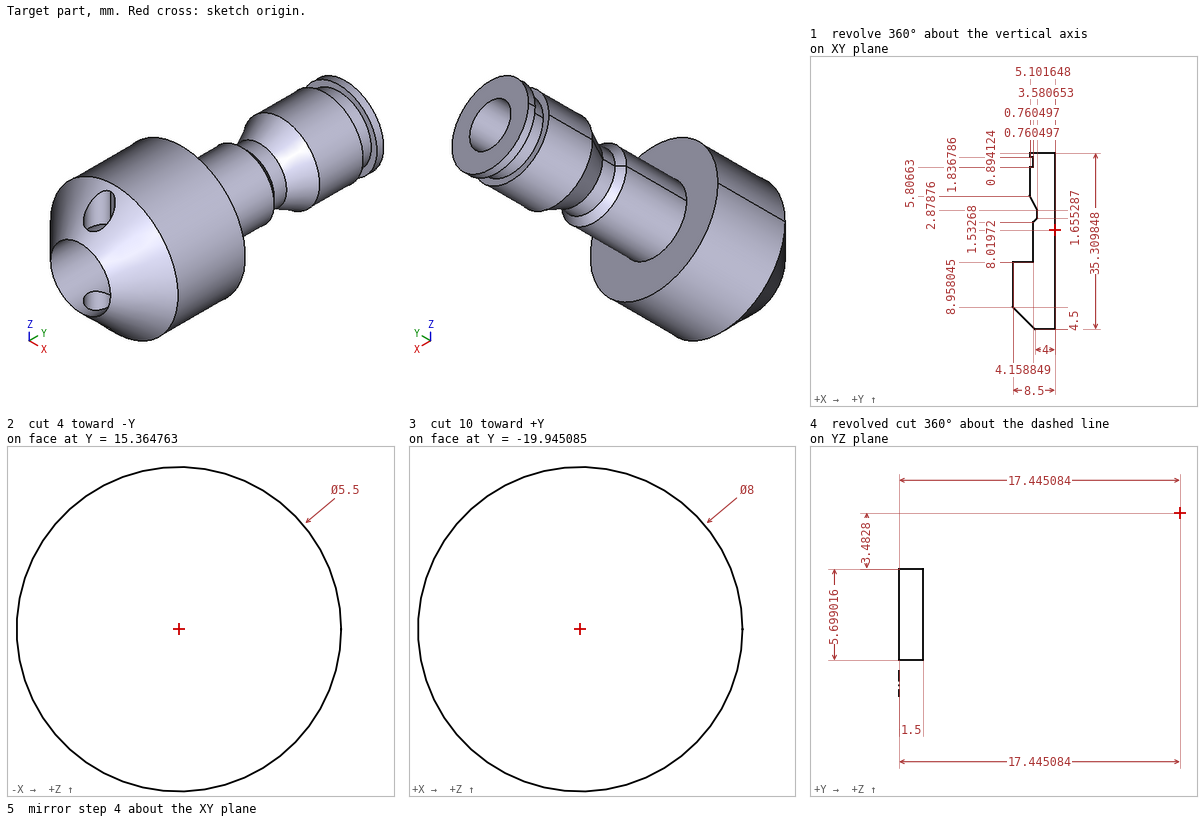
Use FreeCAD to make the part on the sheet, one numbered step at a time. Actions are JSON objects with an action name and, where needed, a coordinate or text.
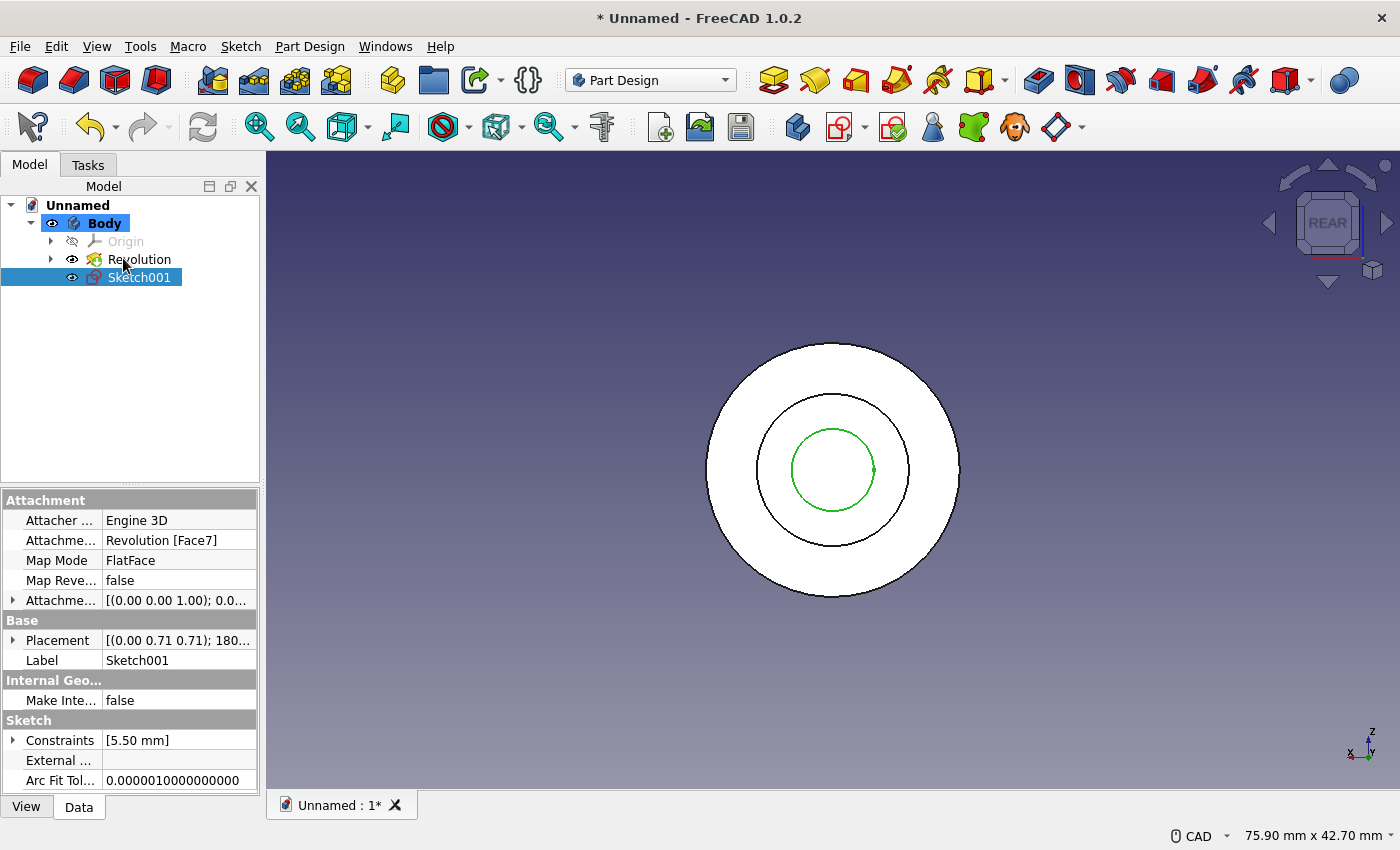
{"action": "left_click", "coordinate": [1039, 80]}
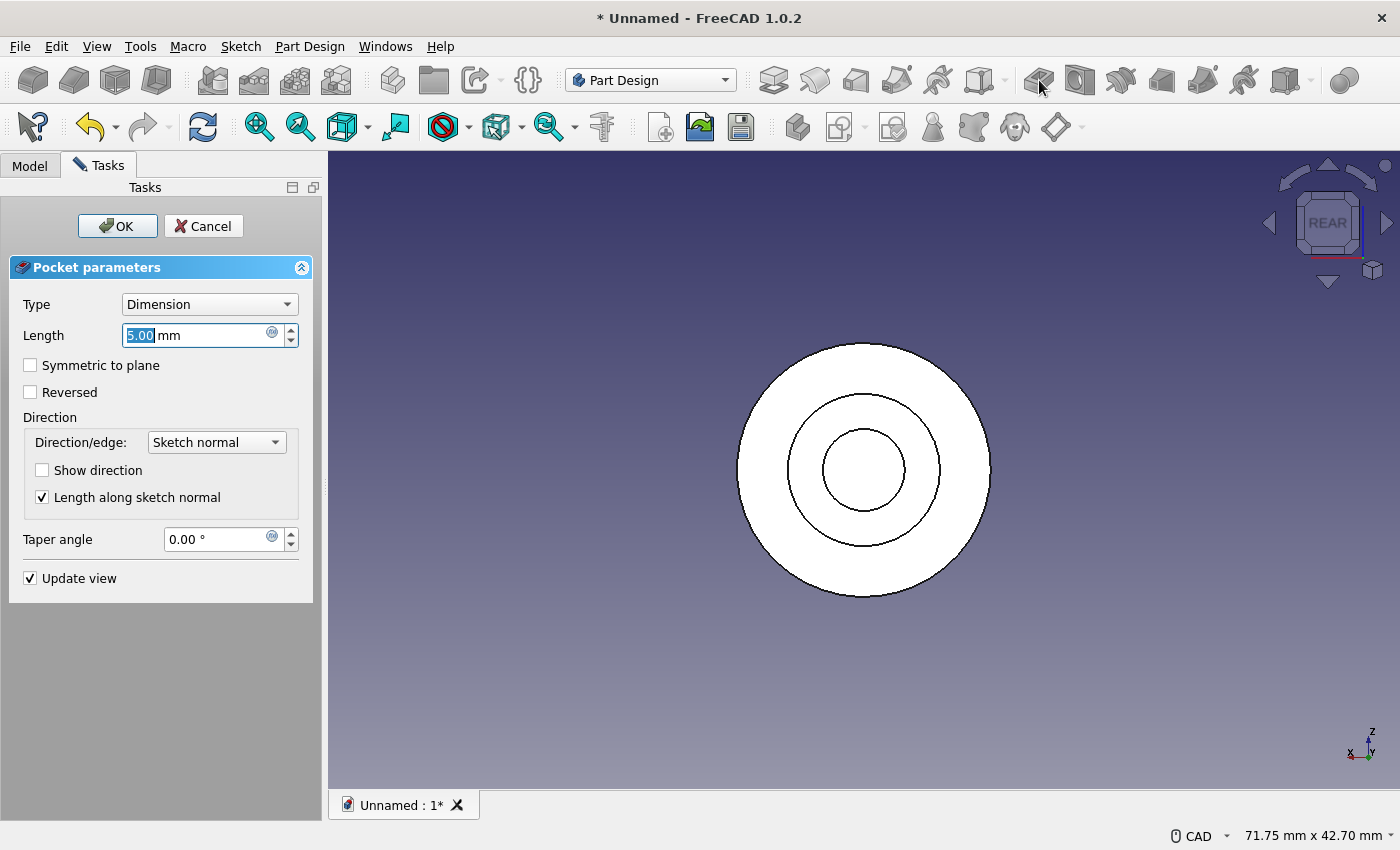
{"action": "type", "text": "4"}
{"action": "key", "text": "Tab"}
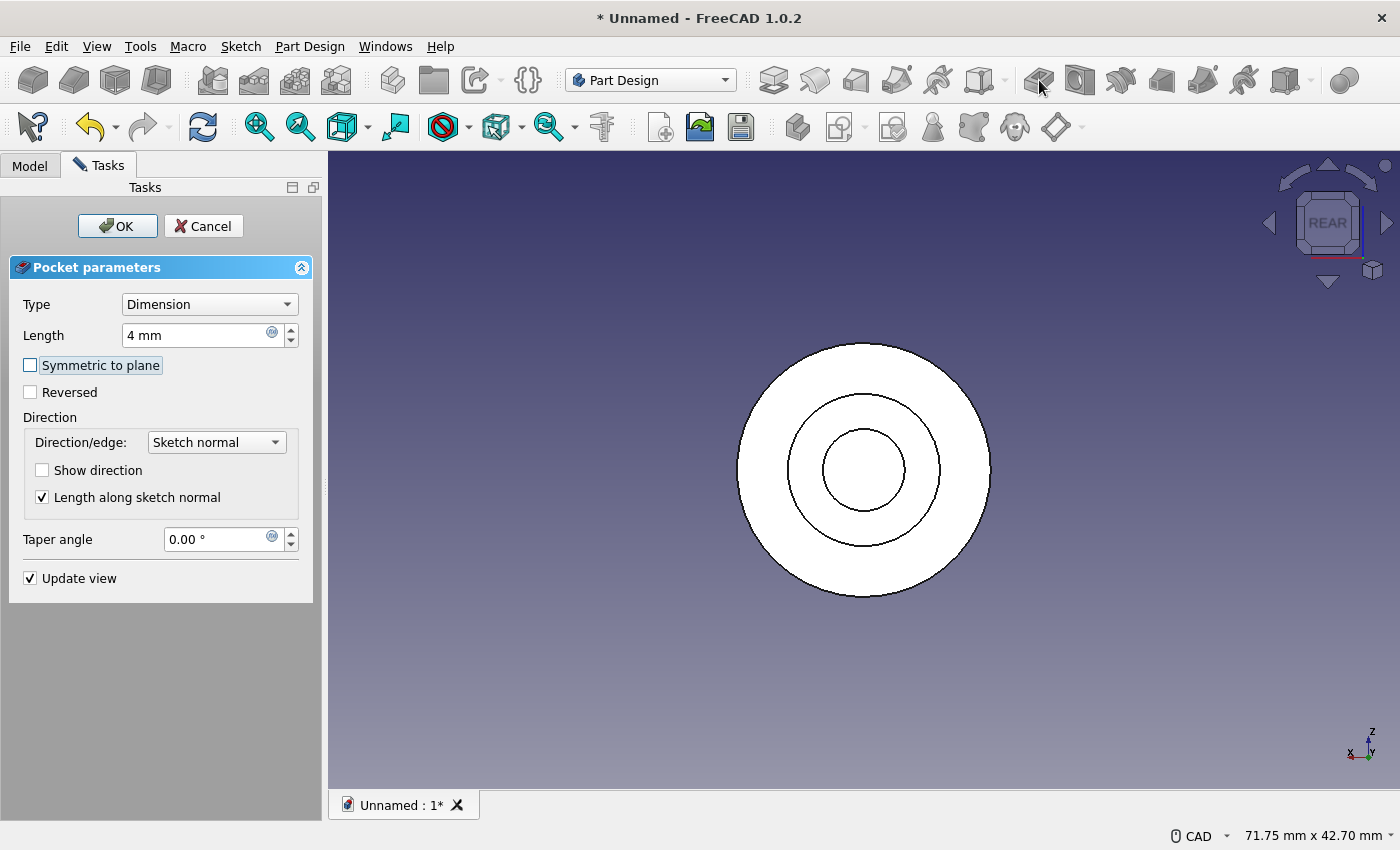
{"action": "left_click", "coordinate": [118, 226]}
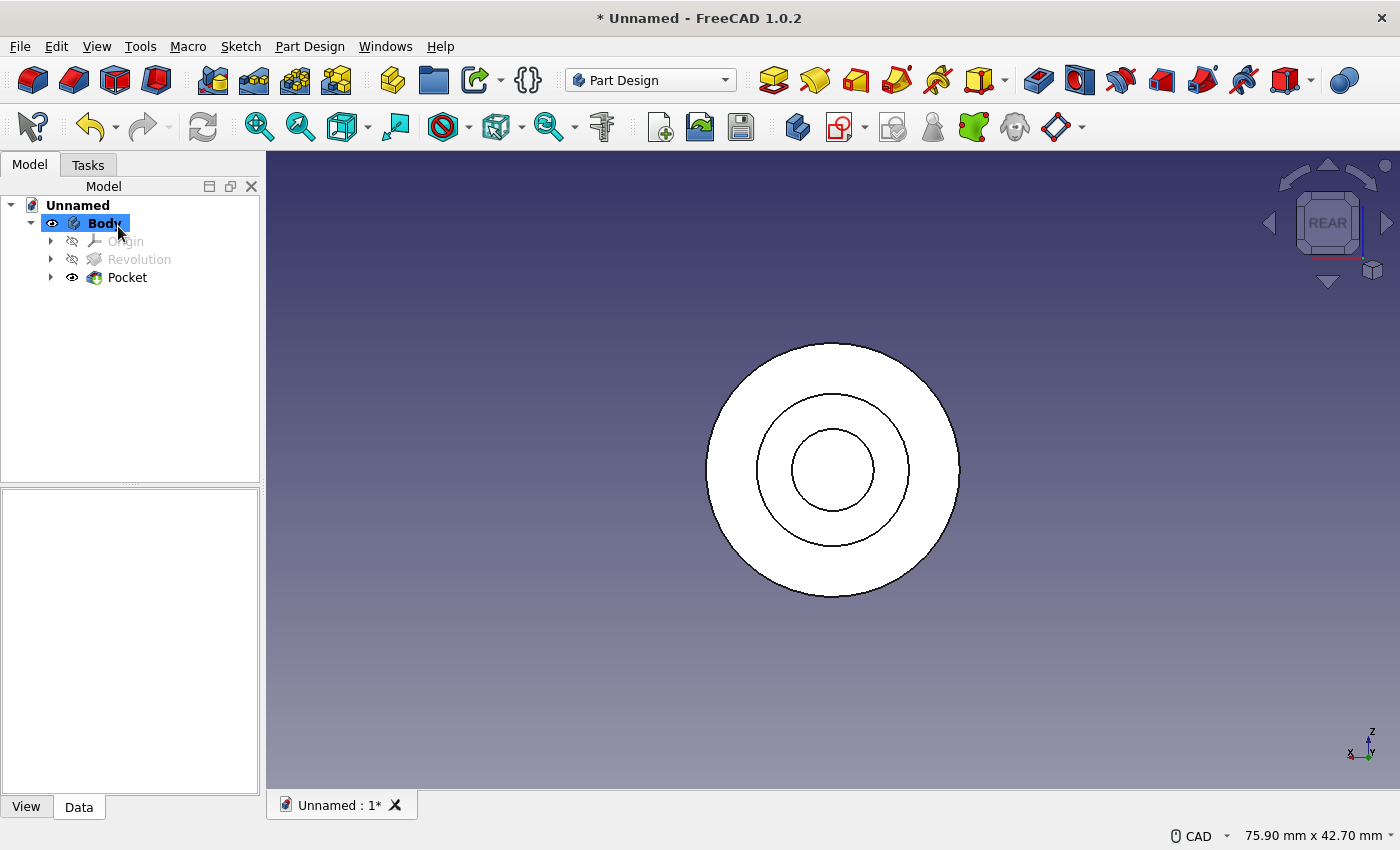
{"action": "key", "text": "v f"}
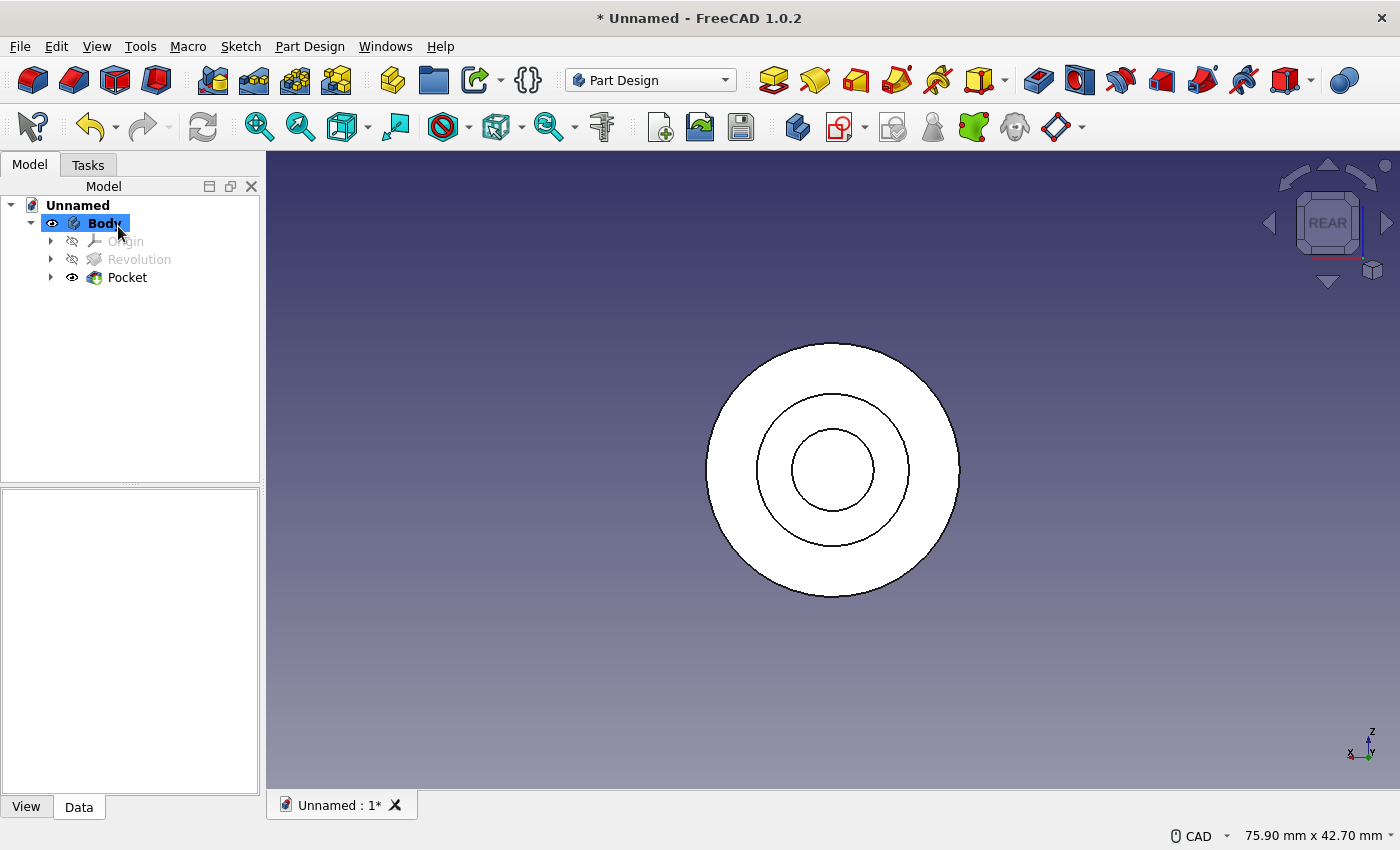
{"action": "key", "text": "0"}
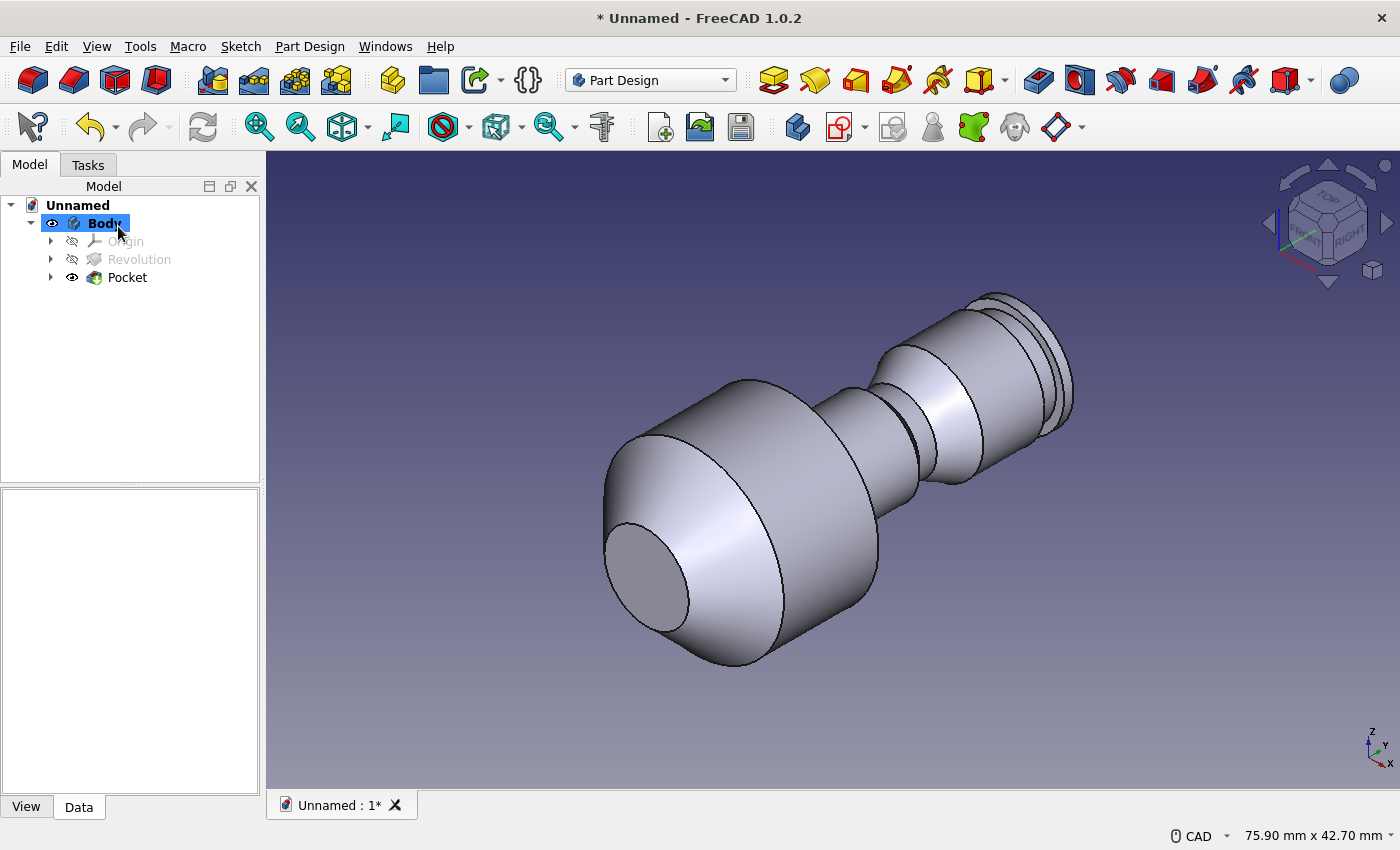
{"action": "left_click", "coordinate": [647, 577]}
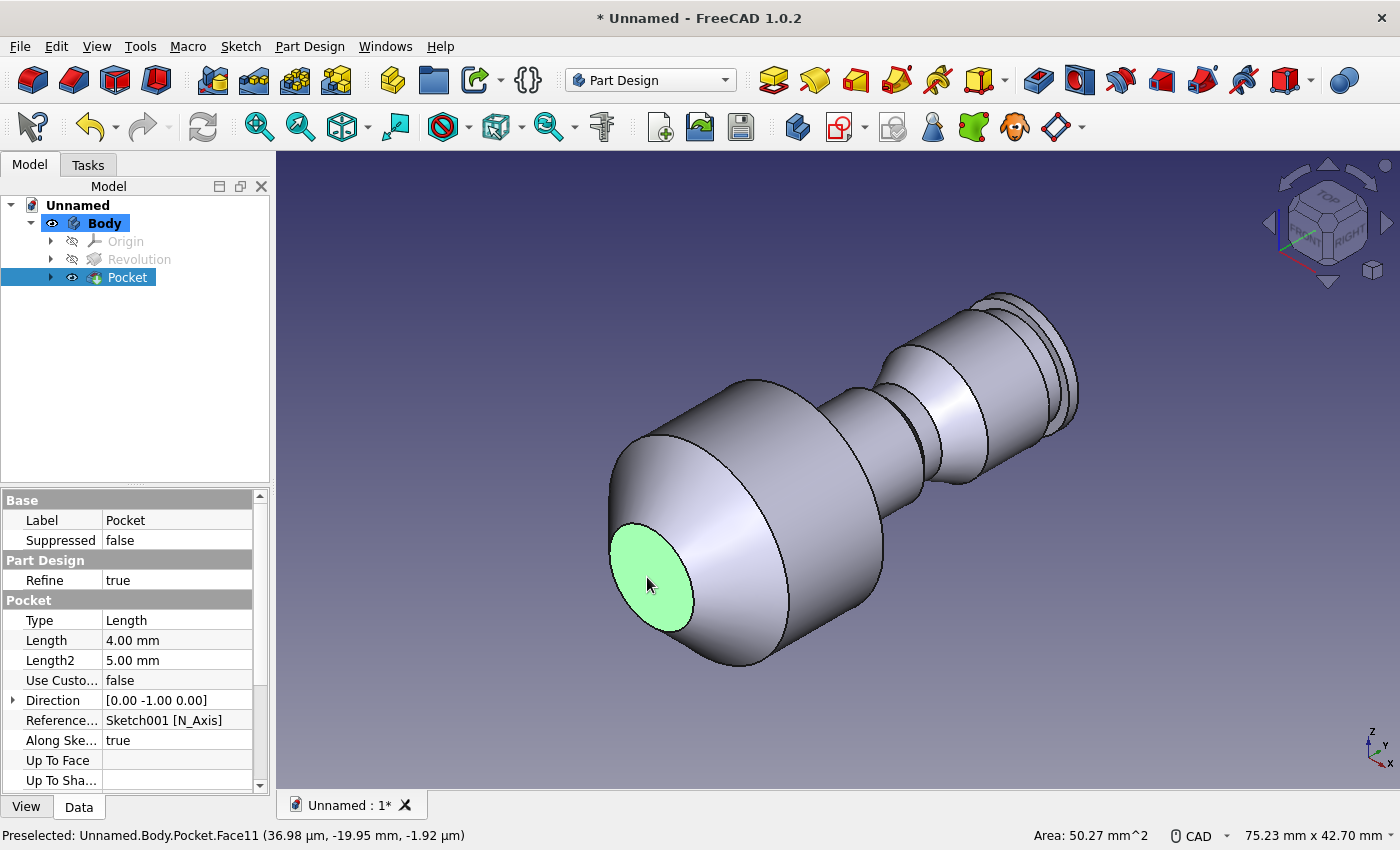
{"action": "left_click", "coordinate": [838, 128]}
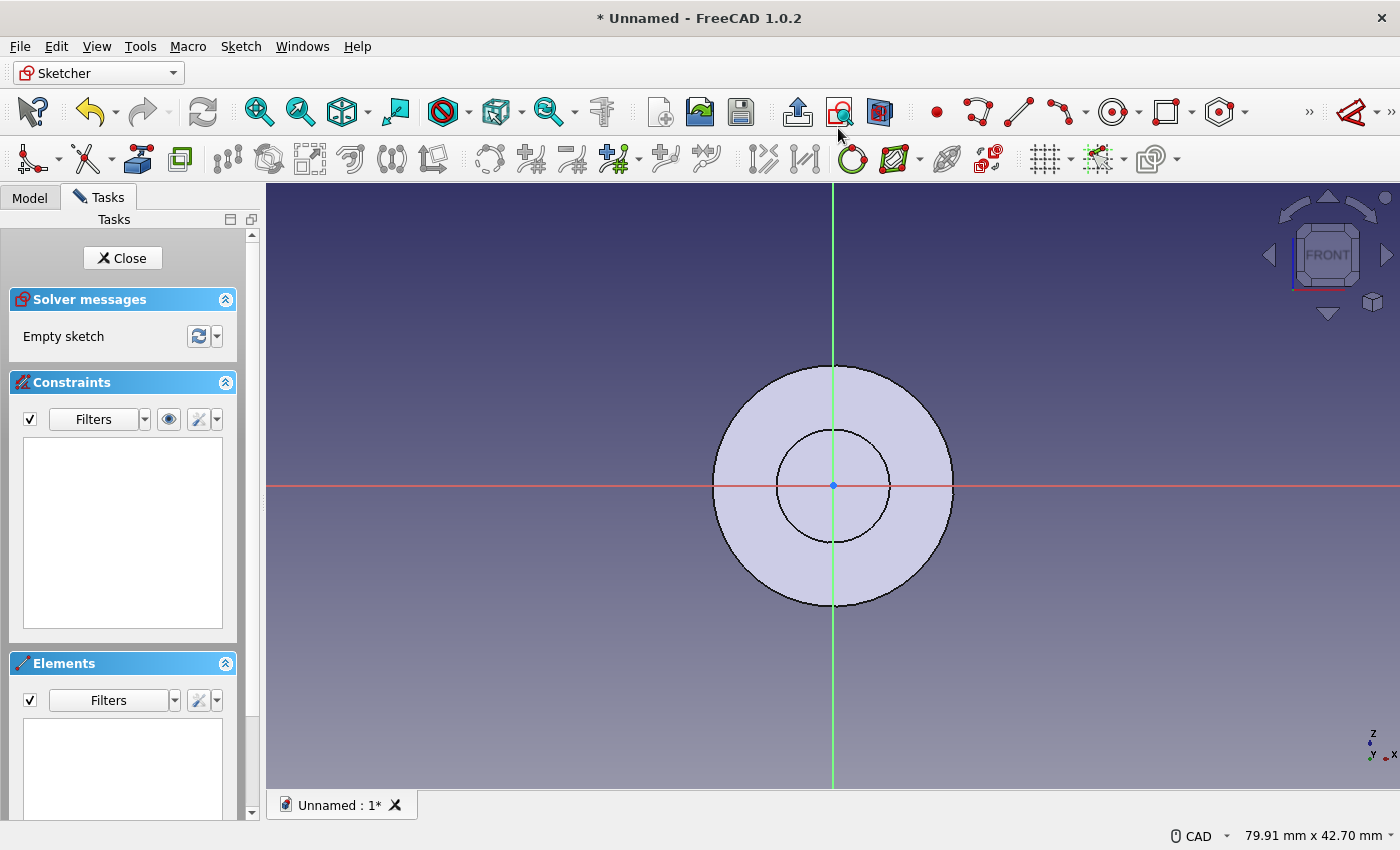
{"action": "scroll", "coordinate": [863, 486], "scroll_direction": "up", "scroll_amount": 6}